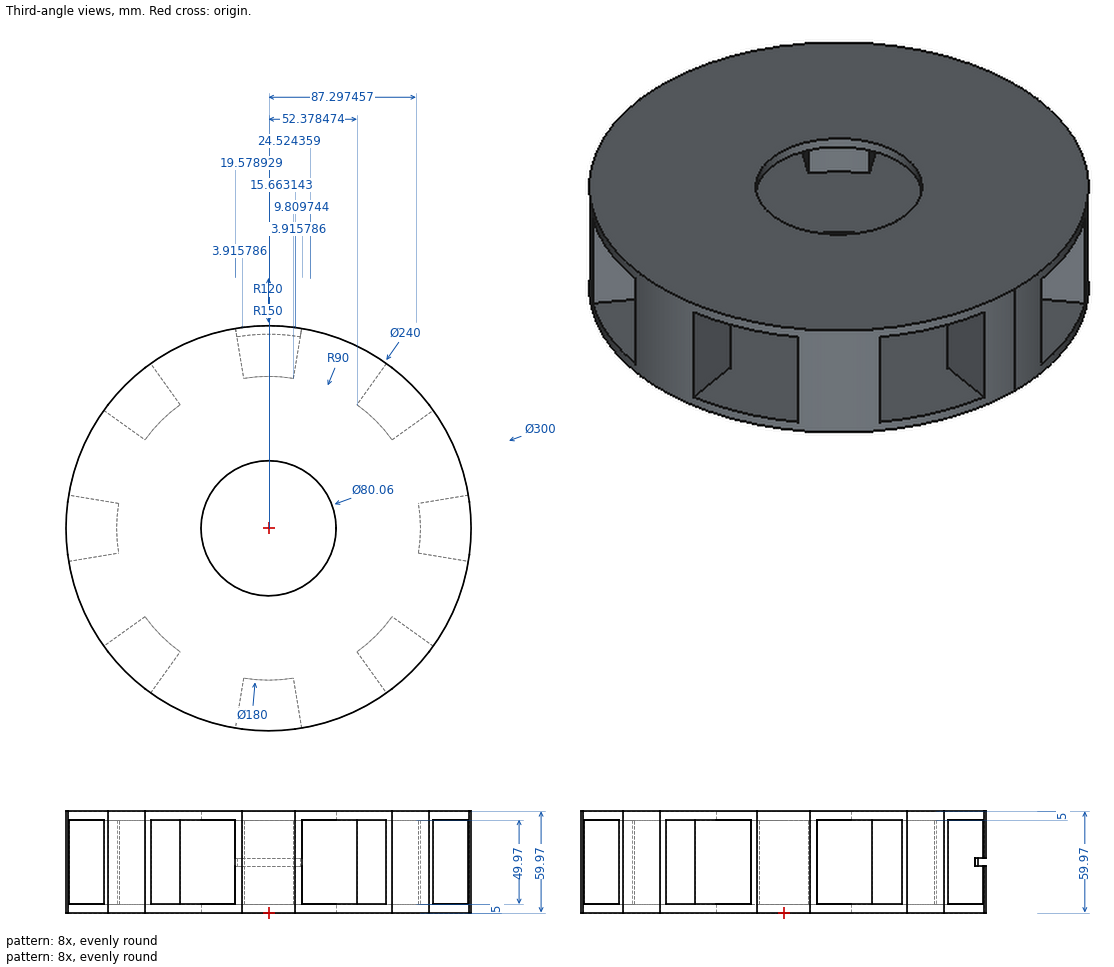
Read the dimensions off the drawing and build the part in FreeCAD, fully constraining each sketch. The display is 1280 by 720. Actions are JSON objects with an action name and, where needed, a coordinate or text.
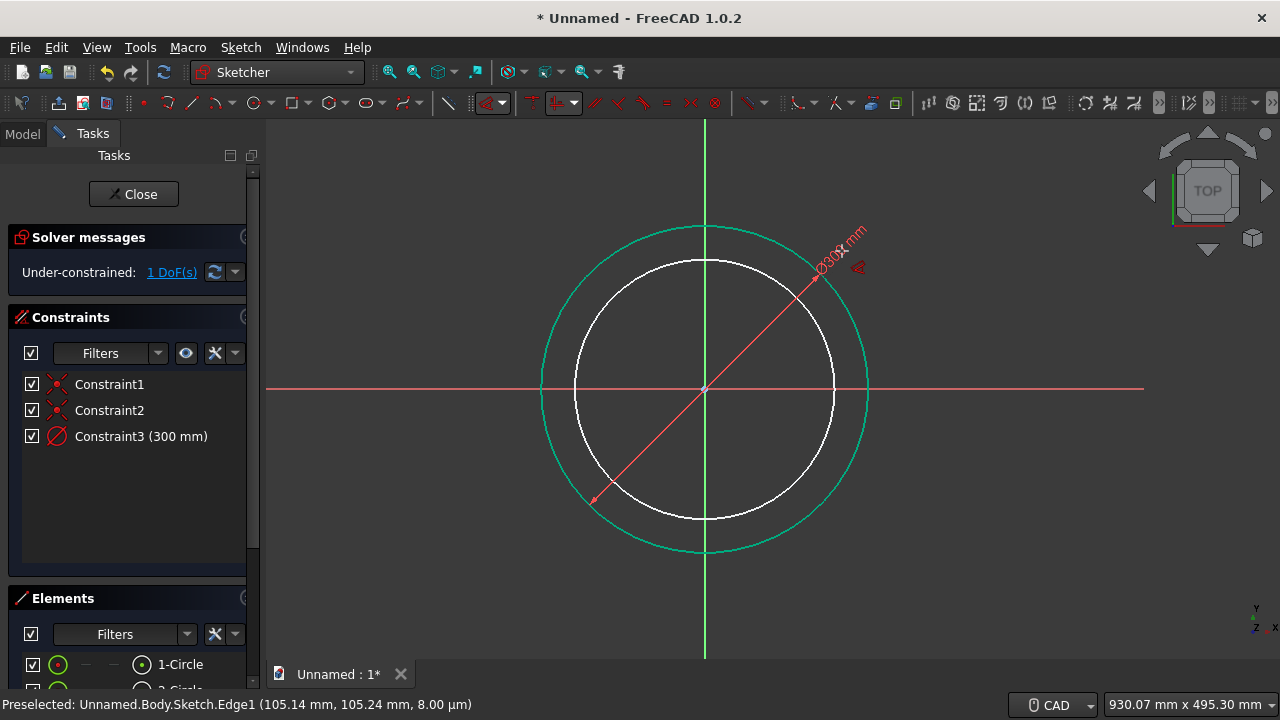
{"action": "left_click", "coordinate": [796, 297]}
{"action": "left_click", "coordinate": [882, 336]}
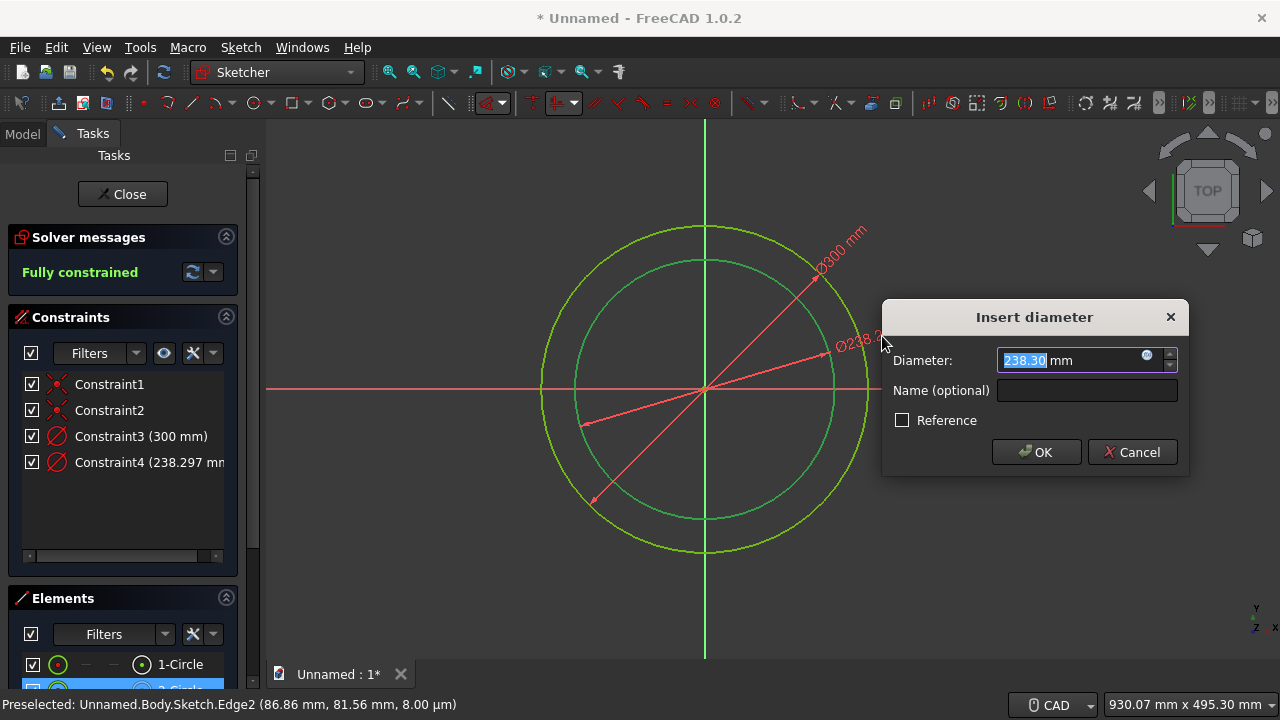
{"action": "type", "text": "240"}
{"action": "key", "text": "Return"}
{"action": "key", "text": "Escape"}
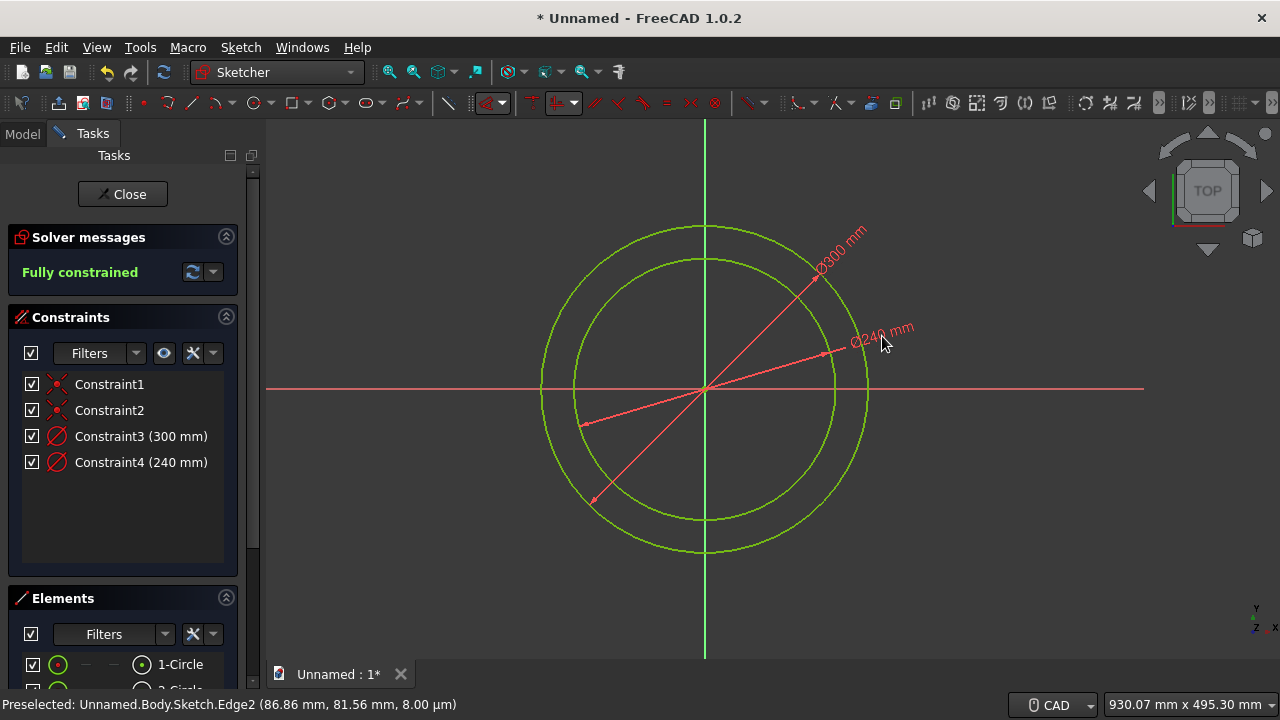
{"action": "left_click", "coordinate": [123, 194]}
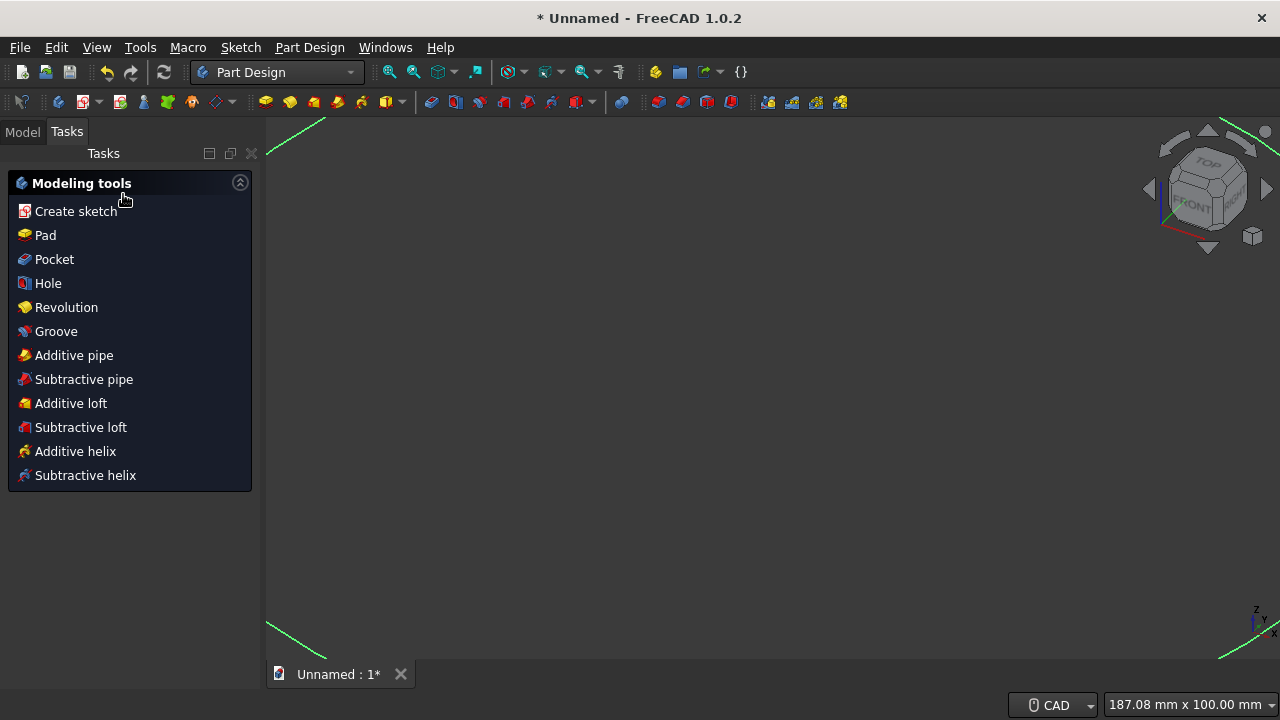
{"action": "left_click", "coordinate": [266, 102]}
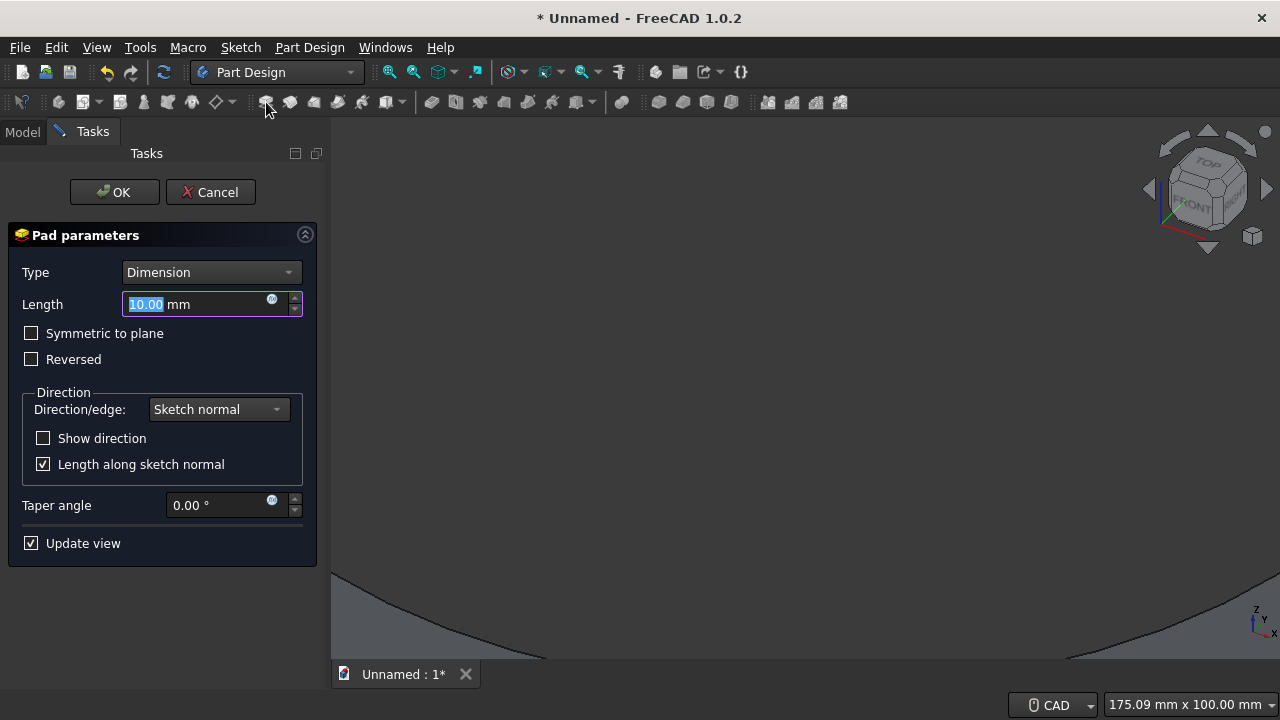
{"action": "type", "text": "59.97"}
{"action": "key", "text": "Tab"}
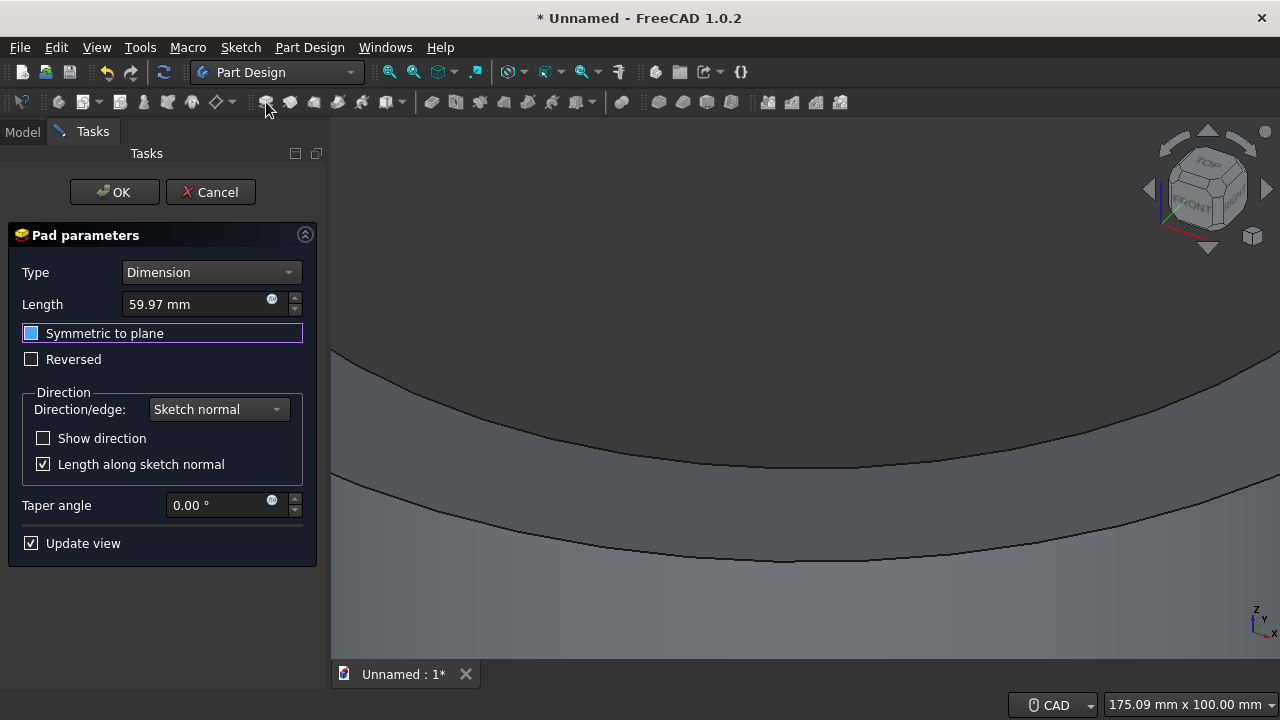
{"action": "left_click", "coordinate": [115, 192]}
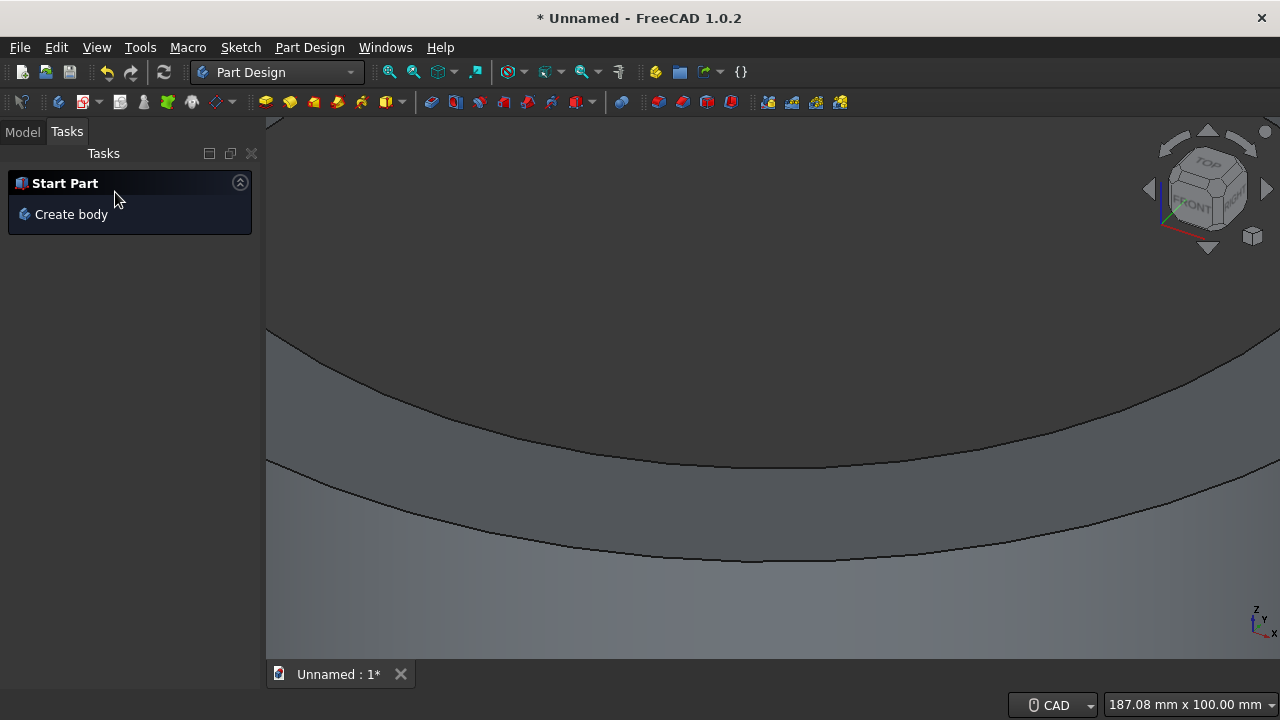
{"action": "key", "text": "v f"}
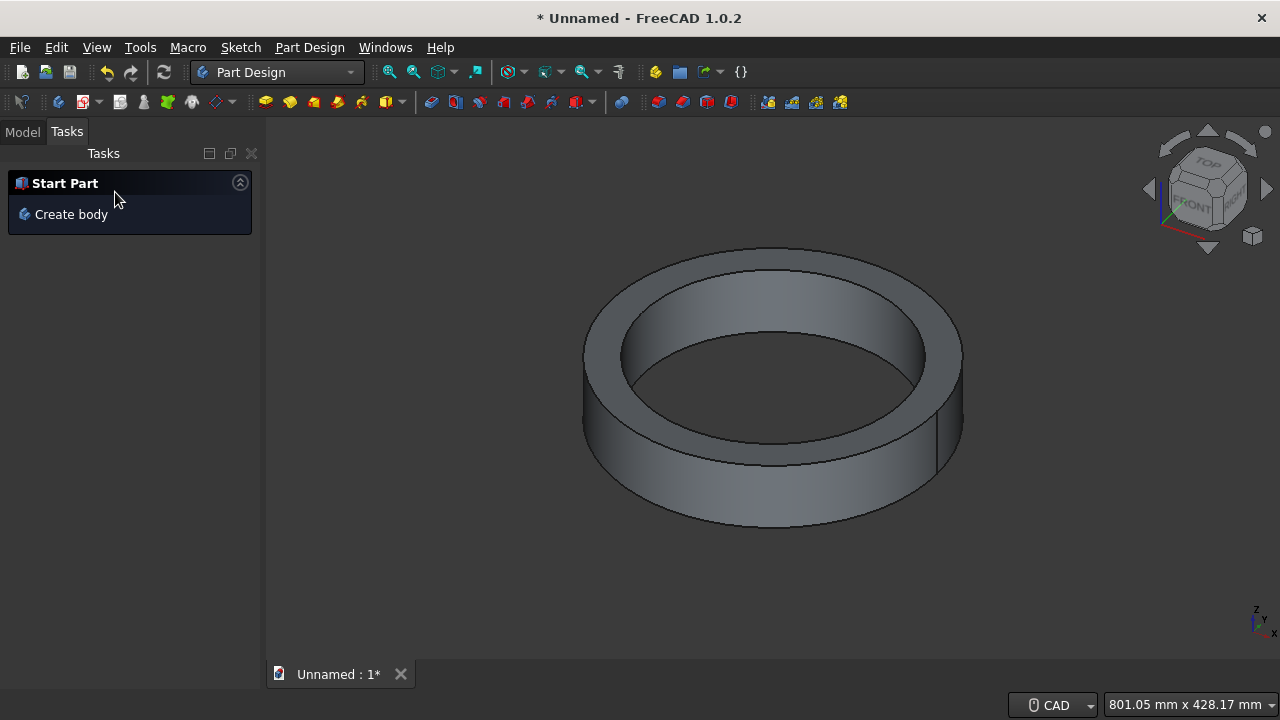
{"action": "key", "text": "5"}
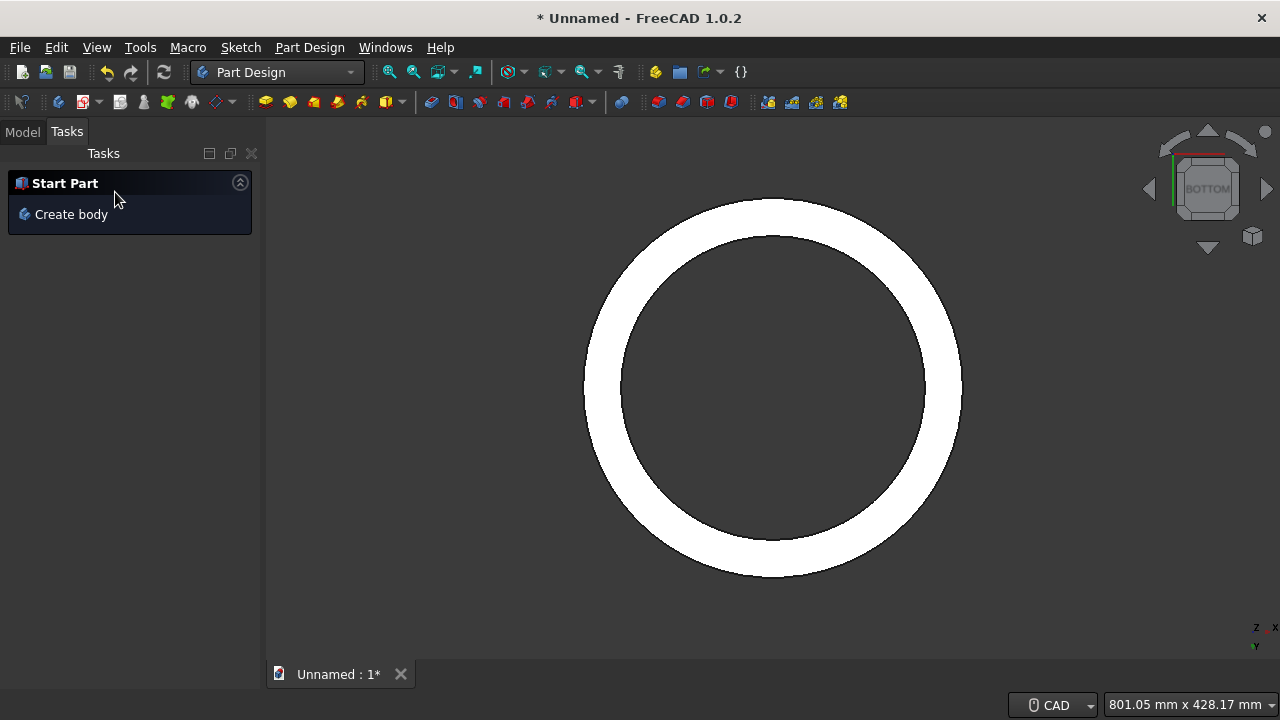
{"action": "left_click", "coordinate": [936, 333]}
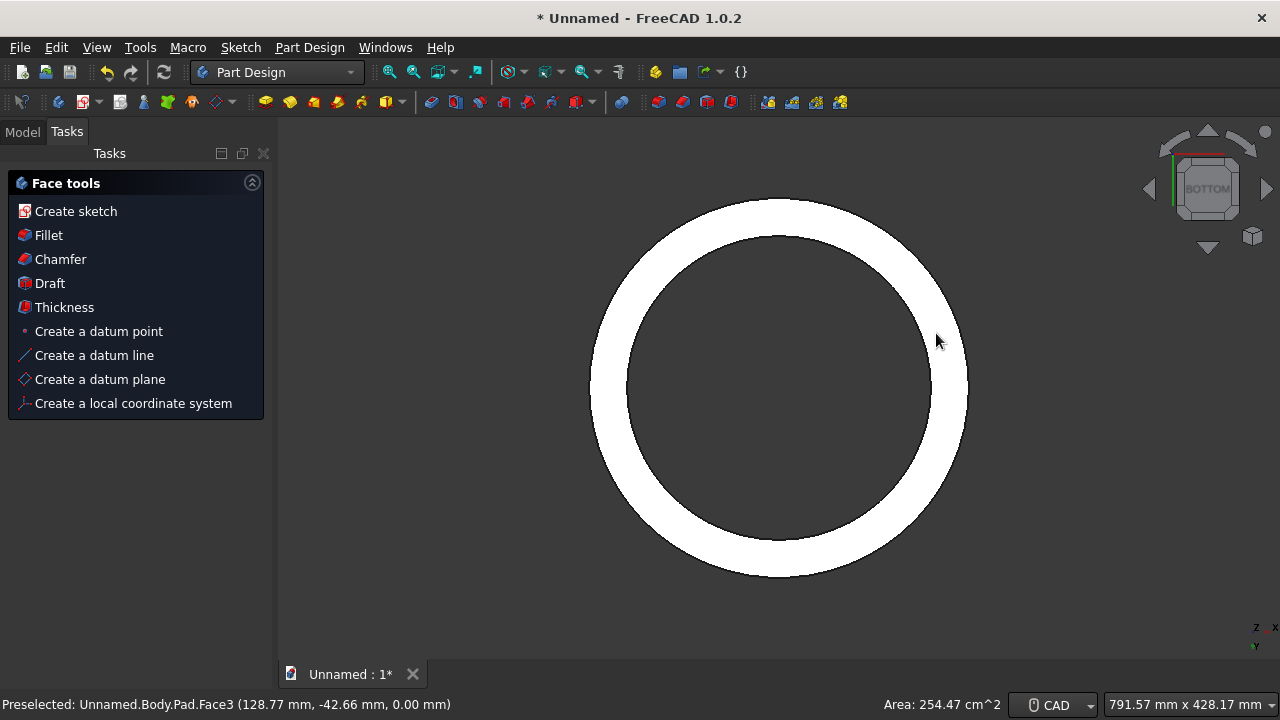
{"action": "left_click", "coordinate": [84, 102]}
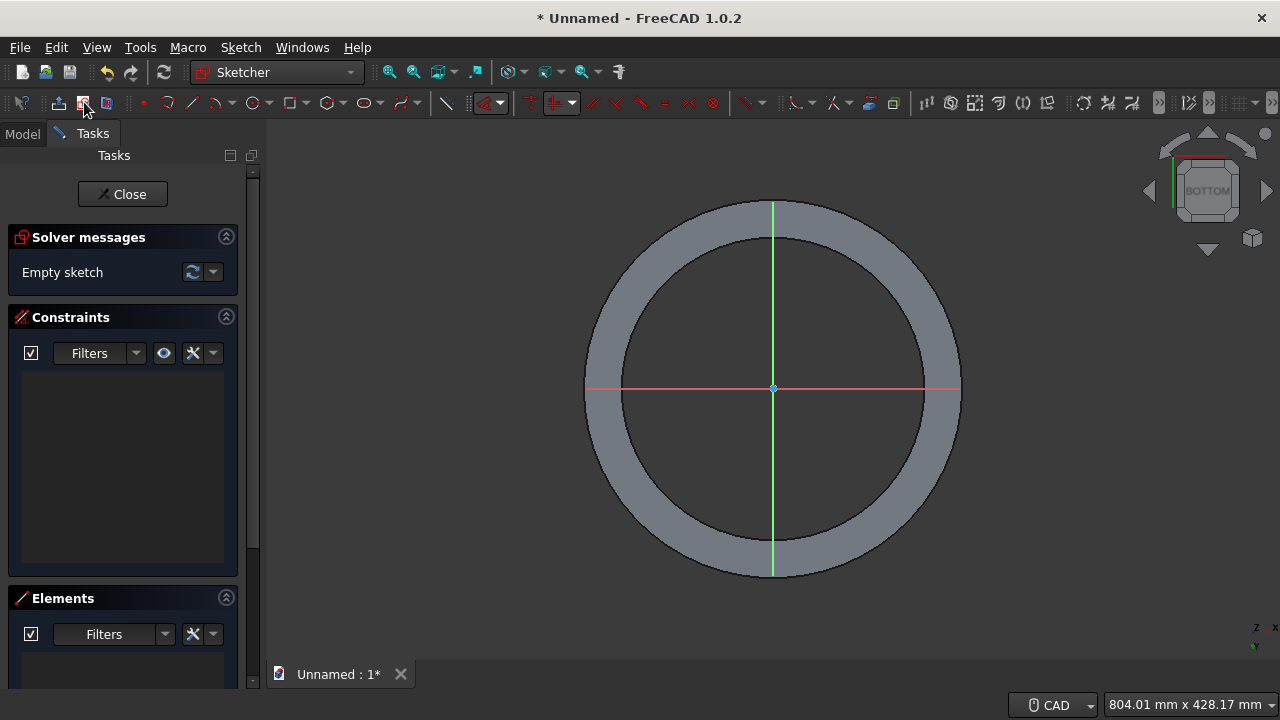
{"action": "left_click", "coordinate": [254, 104]}